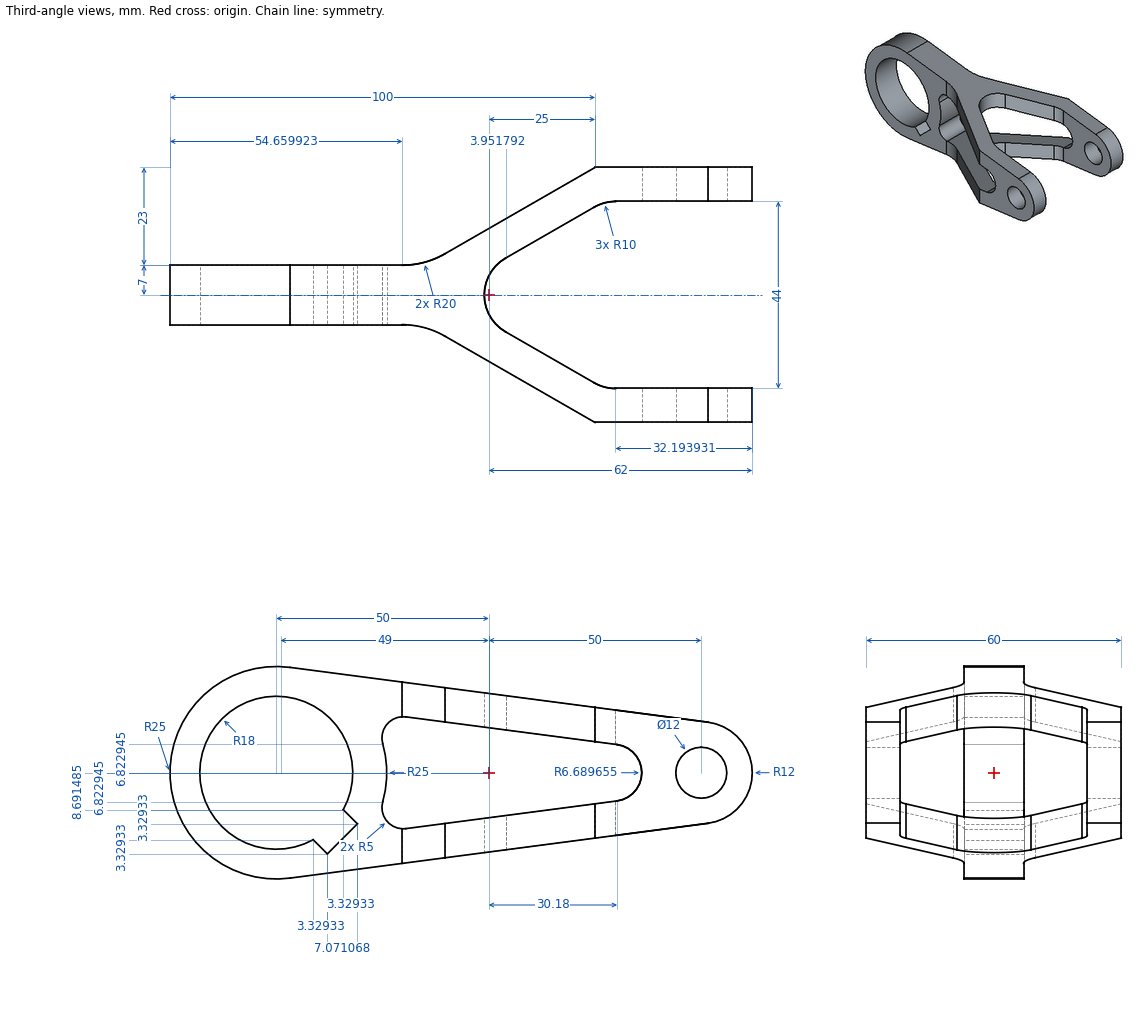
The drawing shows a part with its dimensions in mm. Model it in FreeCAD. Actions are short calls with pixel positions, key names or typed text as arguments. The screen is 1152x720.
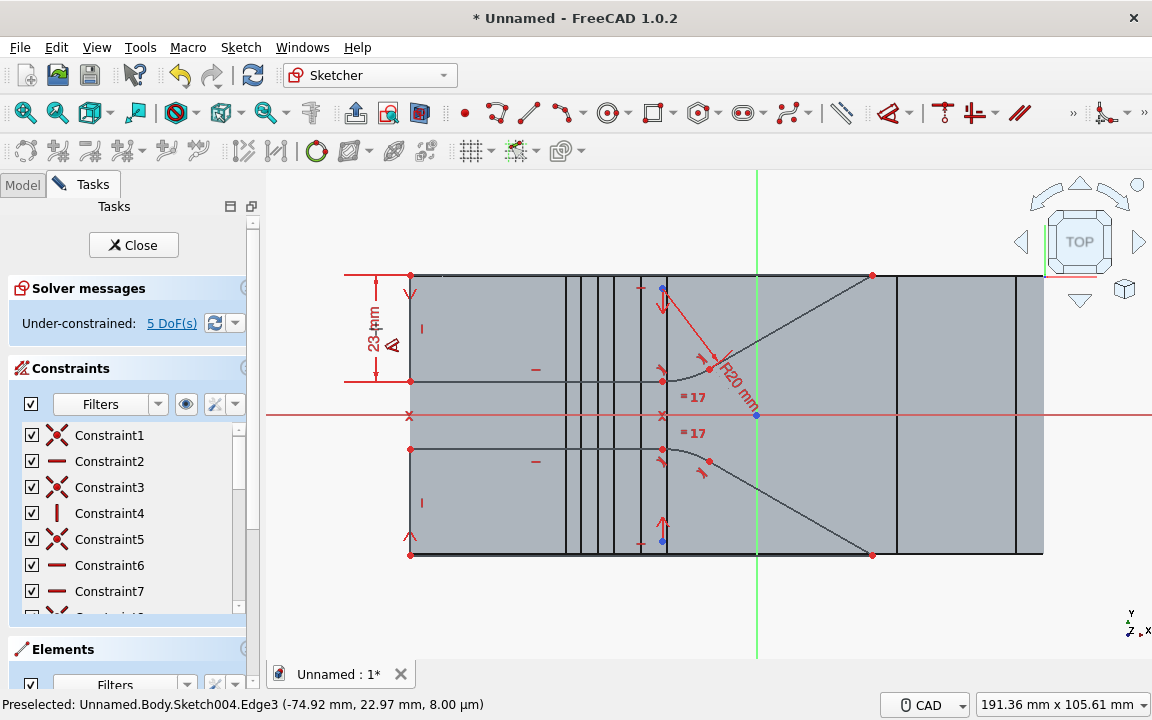
scroll(410, 382, up, 2)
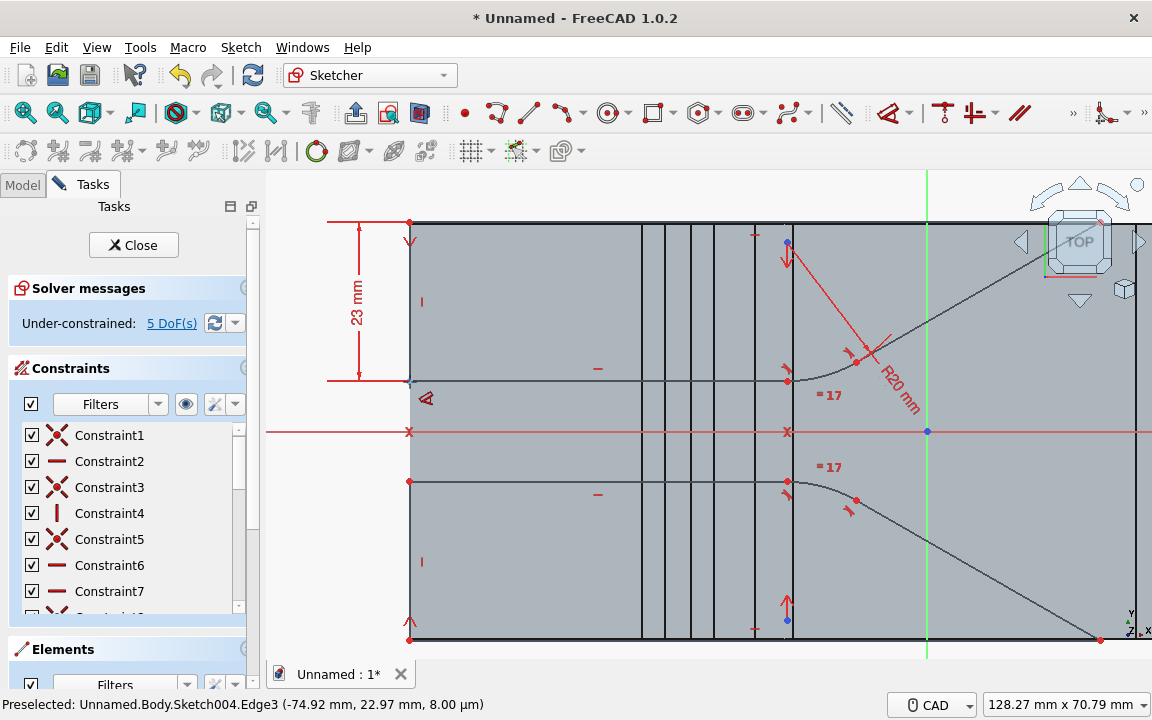
click(410, 381)
click(376, 406)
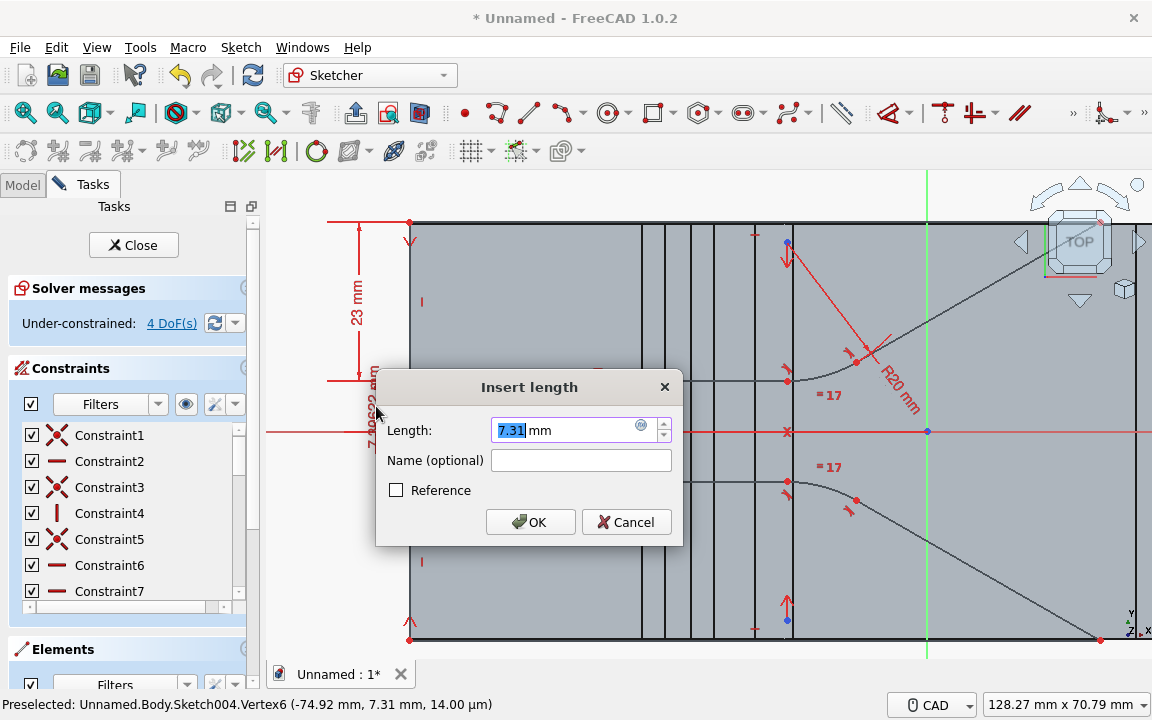
text(7)
key(Return)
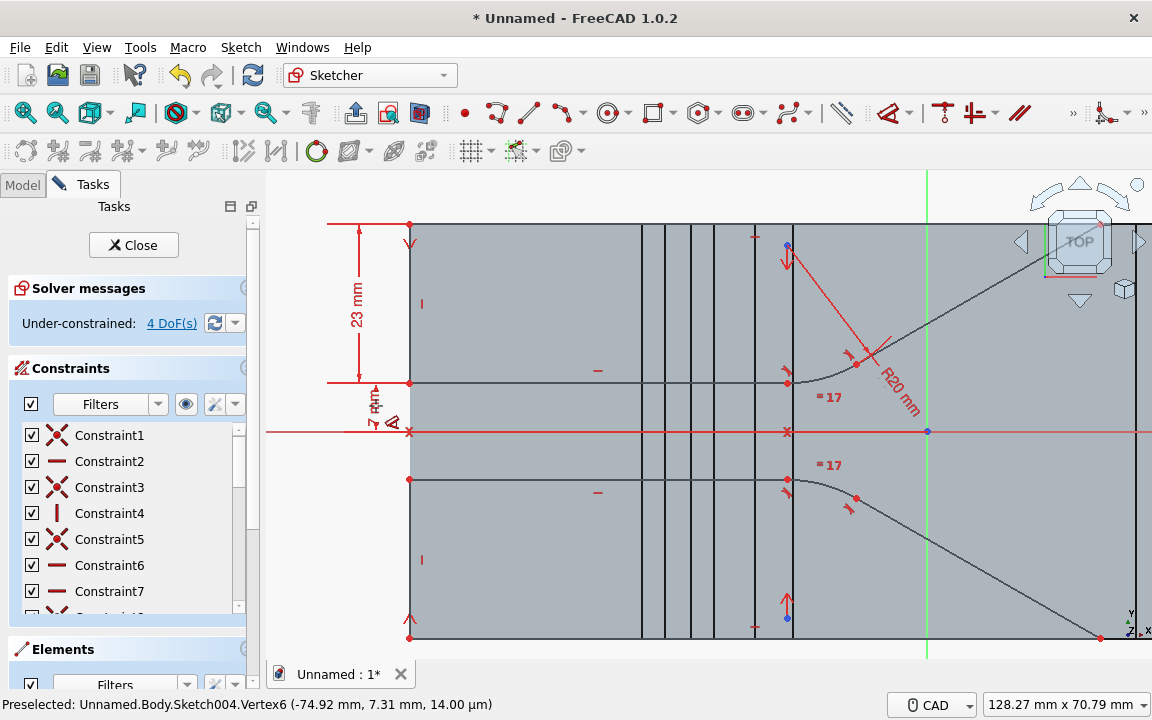
click(893, 224)
click(698, 258)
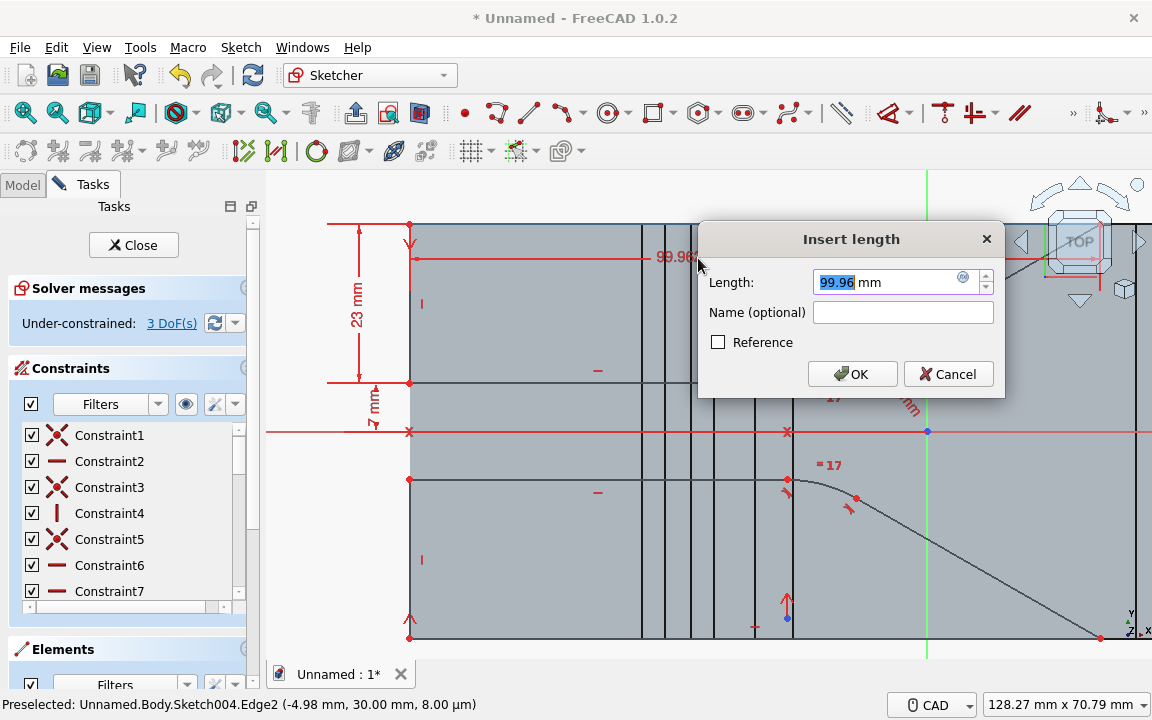
text(100)
key(Return)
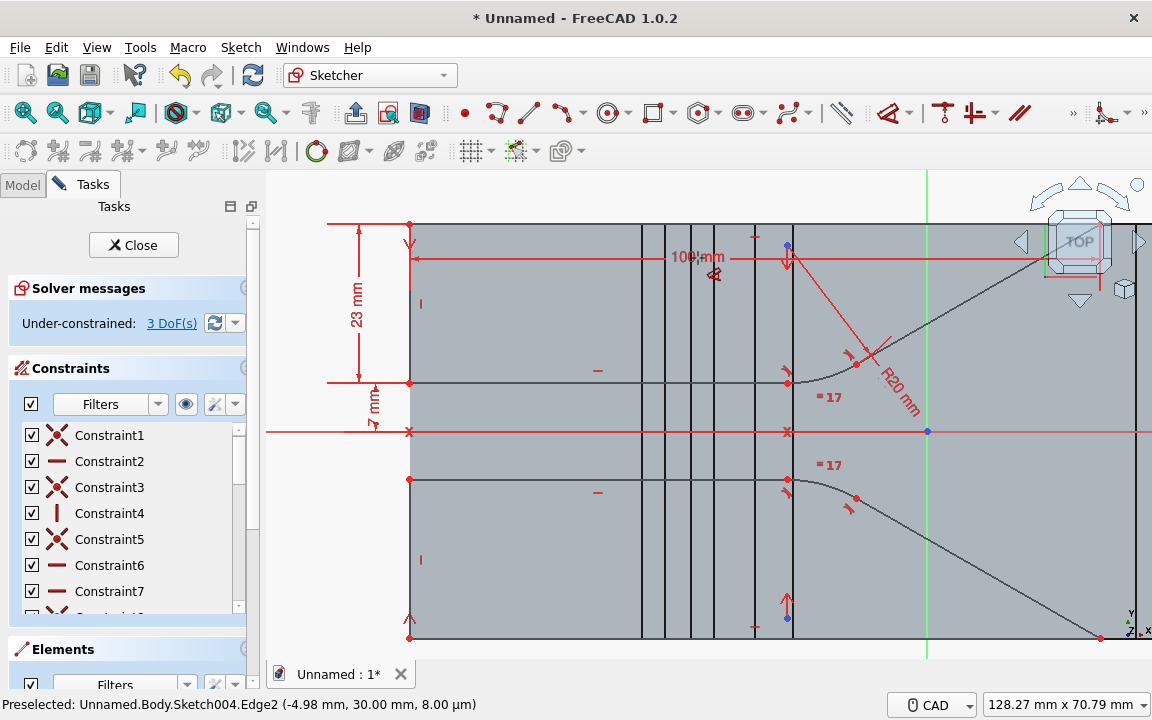
scroll(408, 380, down, 2)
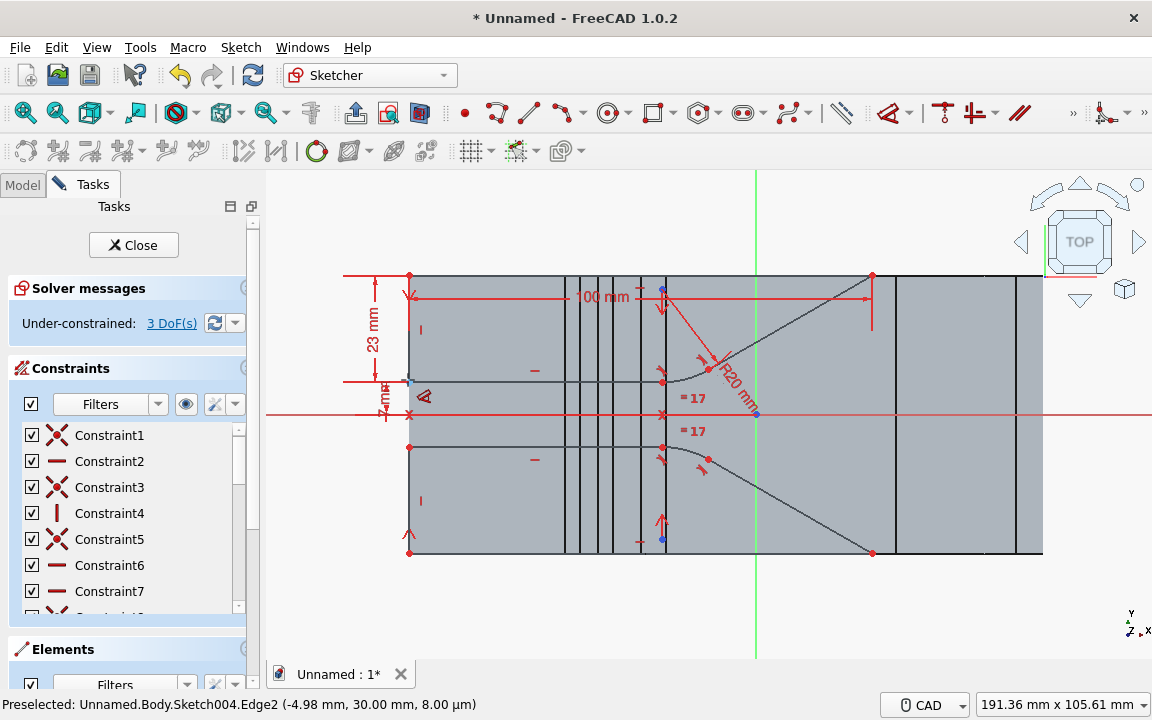
click(548, 554)
click(641, 588)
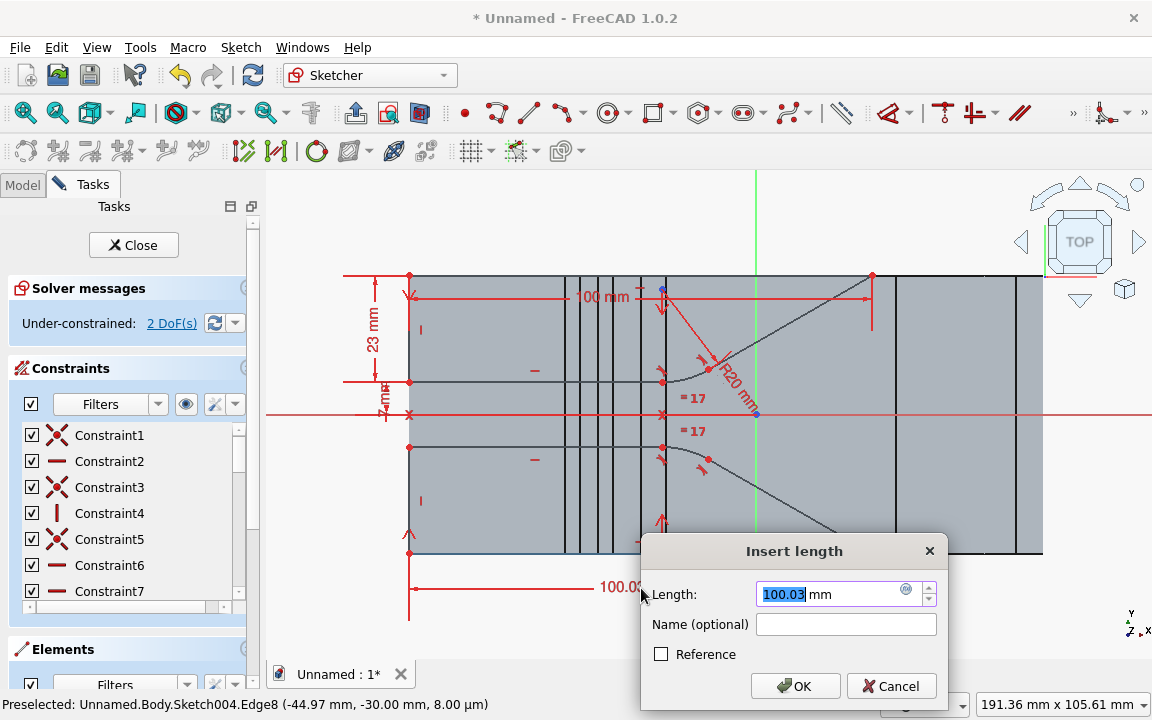
text(100)
key(Return)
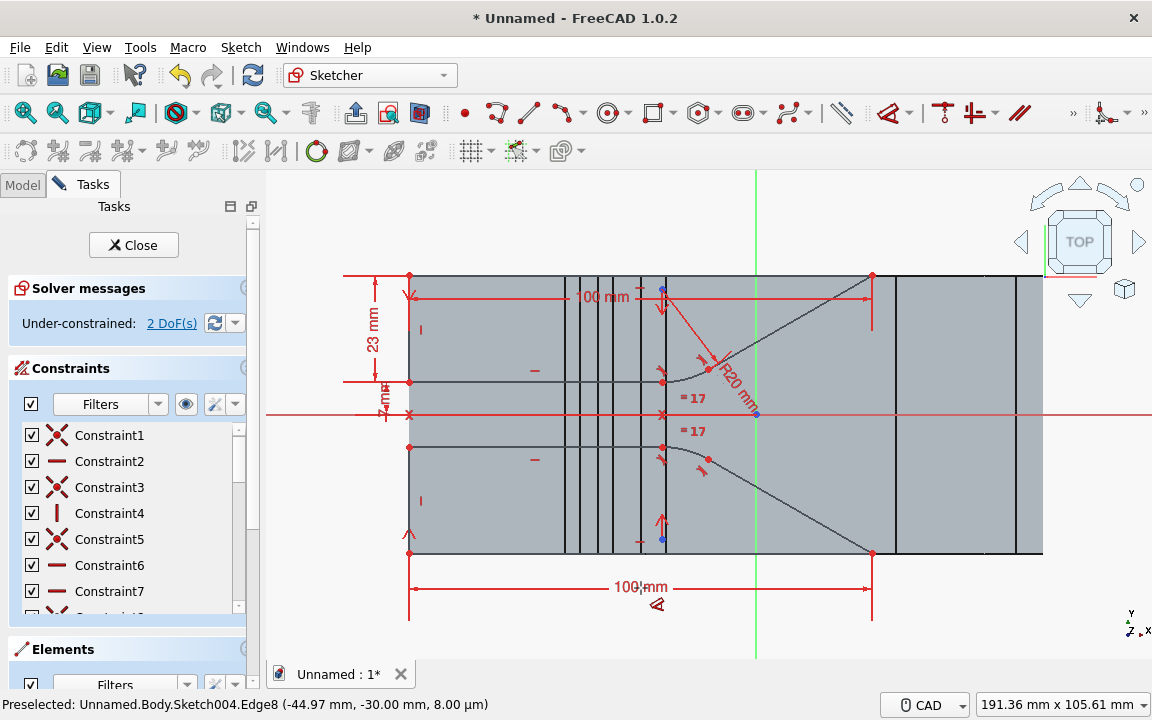
click(872, 276)
click(814, 242)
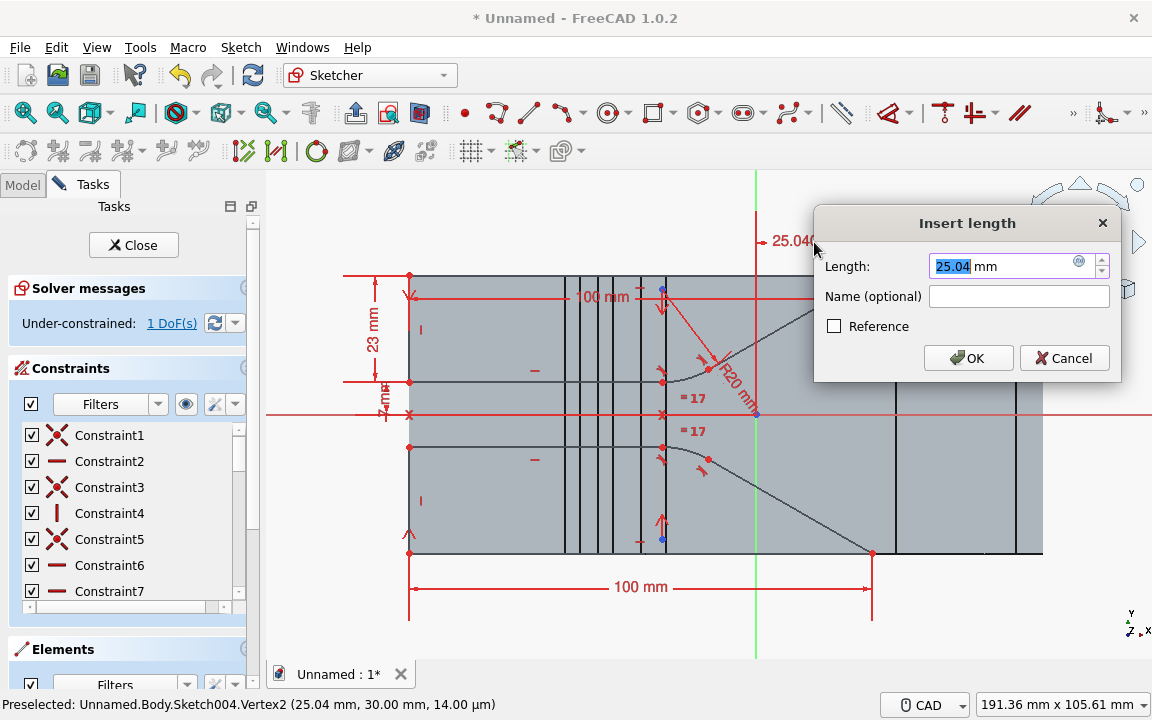
text(25)
key(Return)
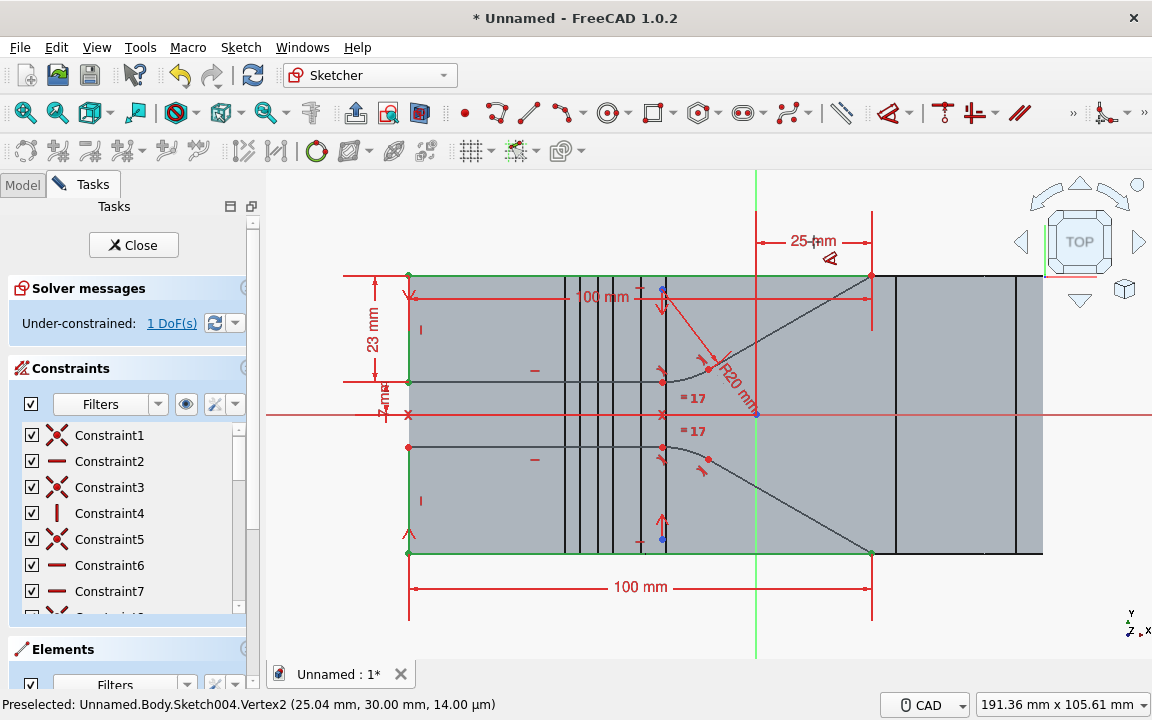
click(485, 382)
click(536, 348)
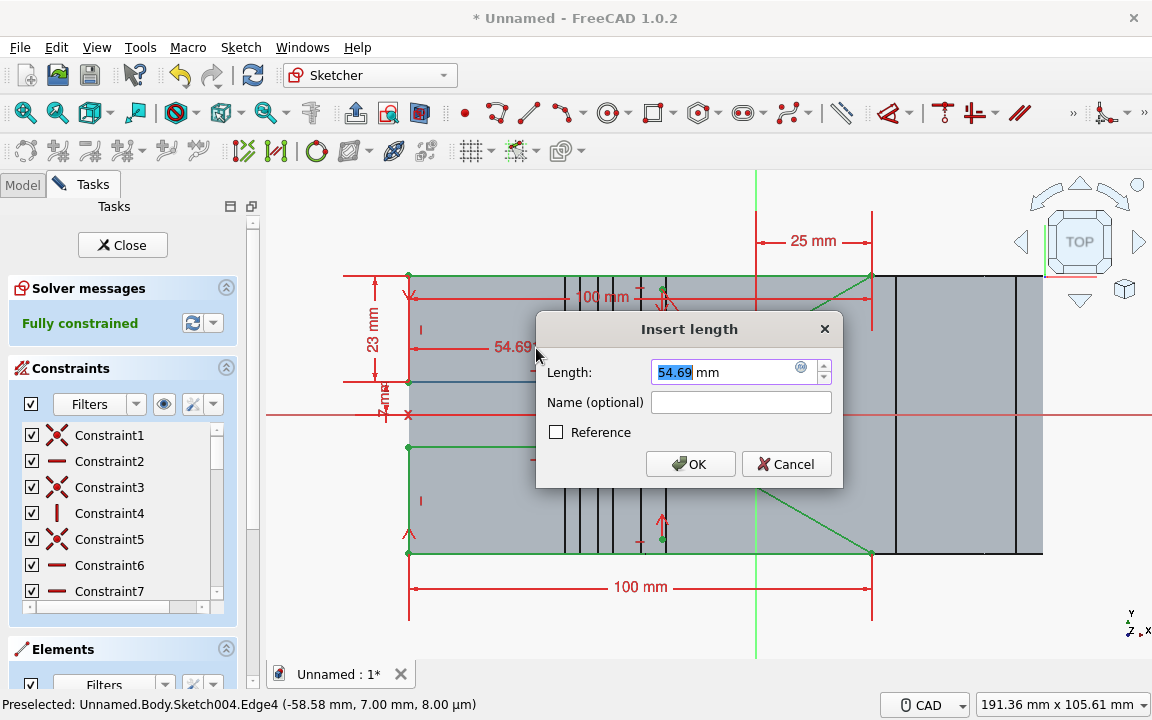
text(54.659923)
key(Return)
key(Escape)